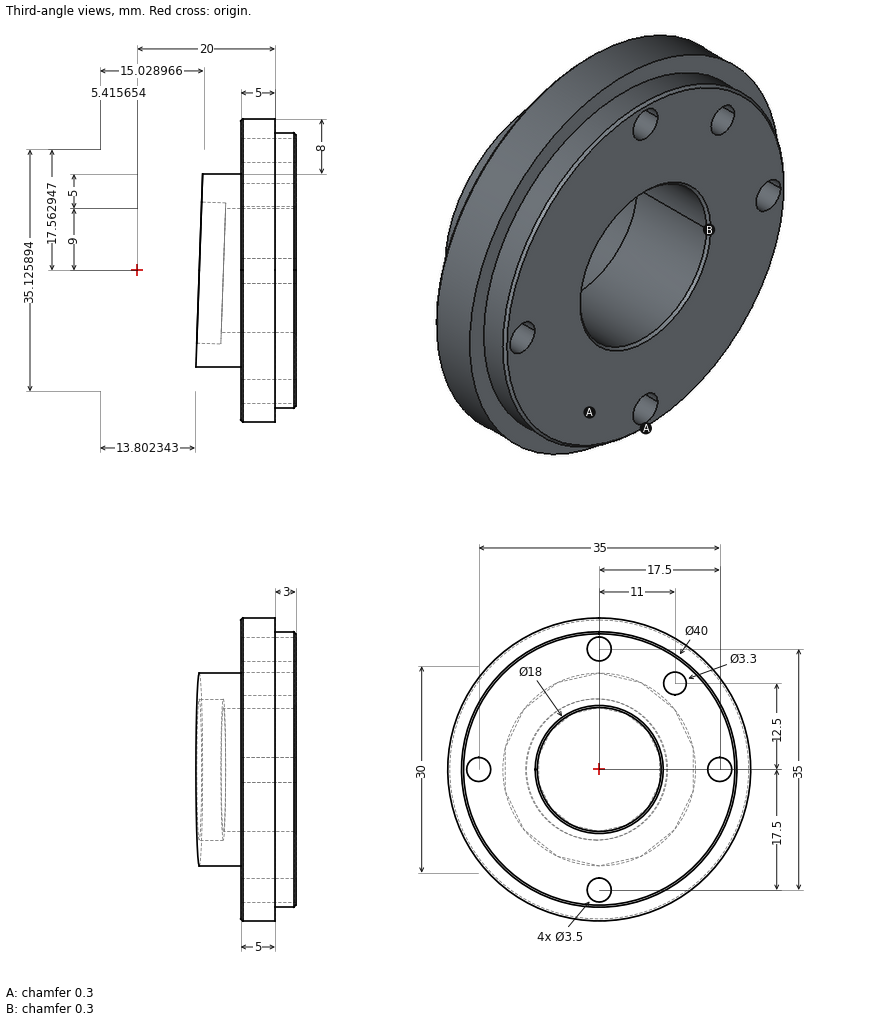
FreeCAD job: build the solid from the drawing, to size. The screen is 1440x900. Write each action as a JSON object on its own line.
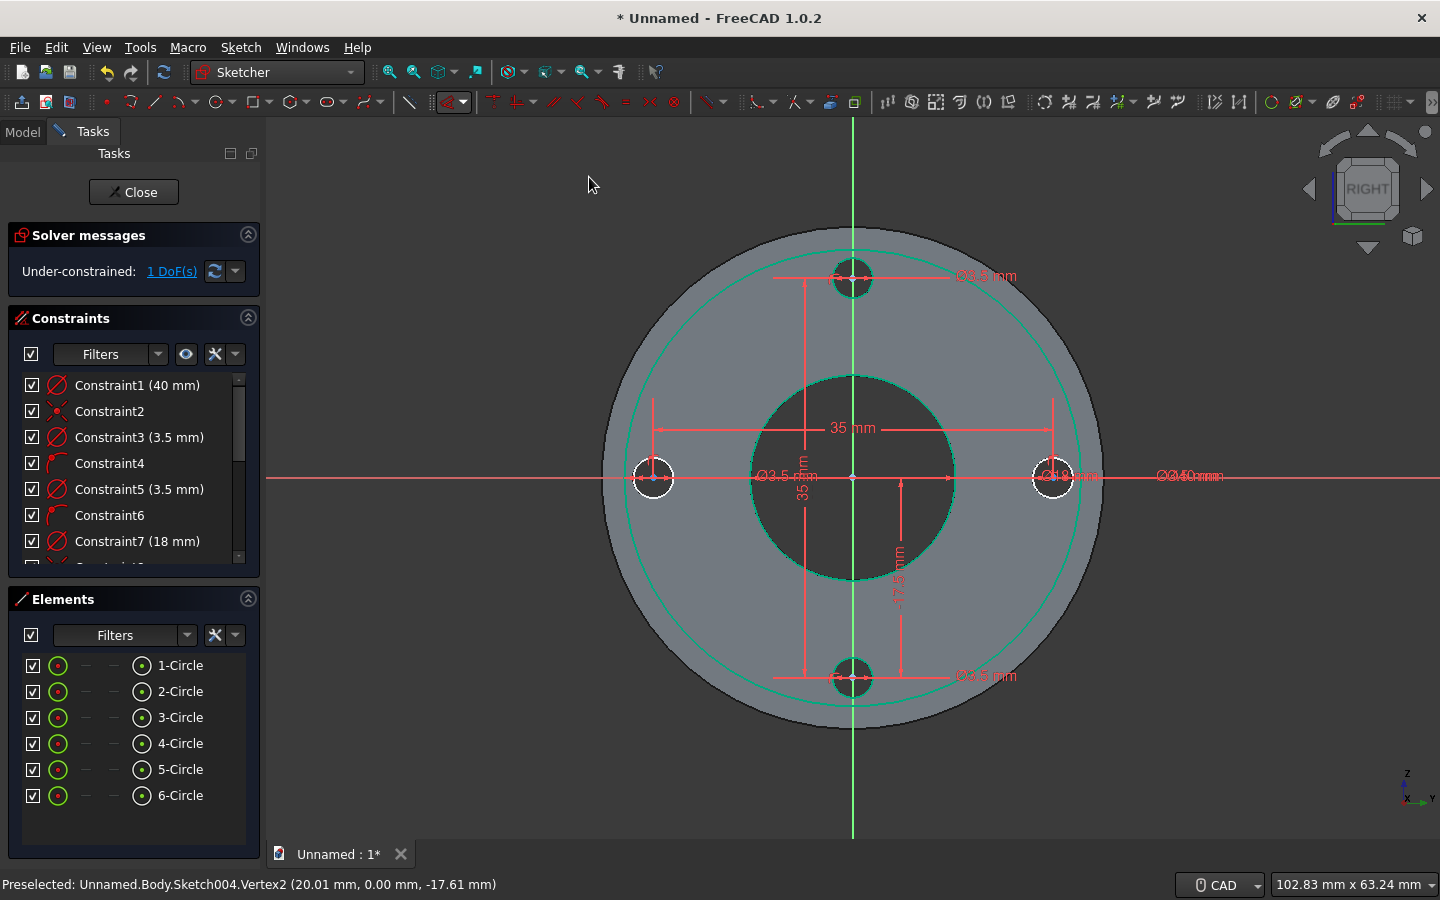
{"action": "left_click", "coordinate": [1053, 478]}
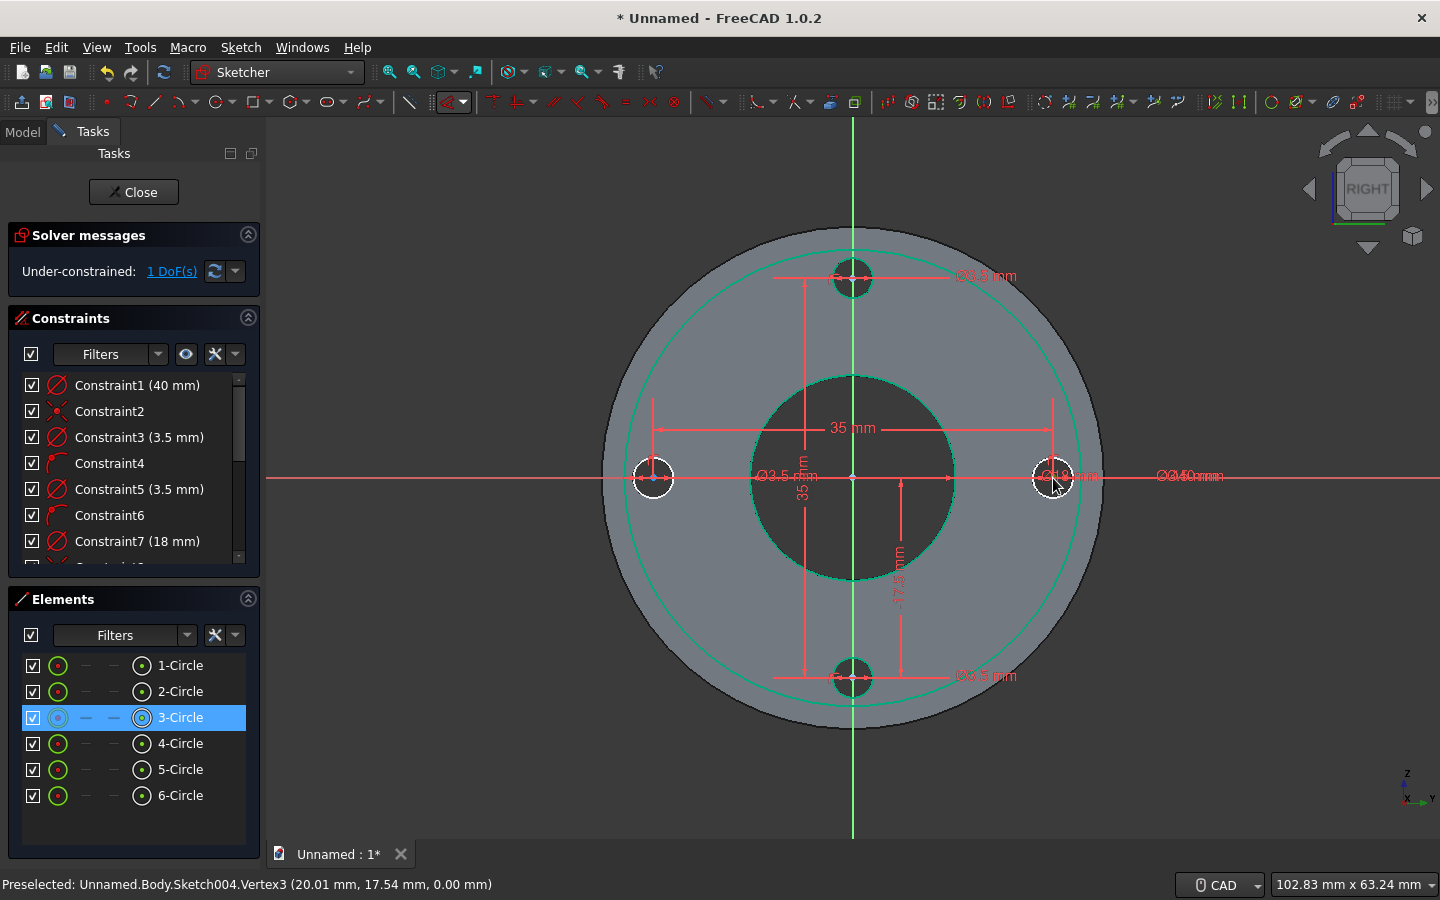
{"action": "key", "text": "l"}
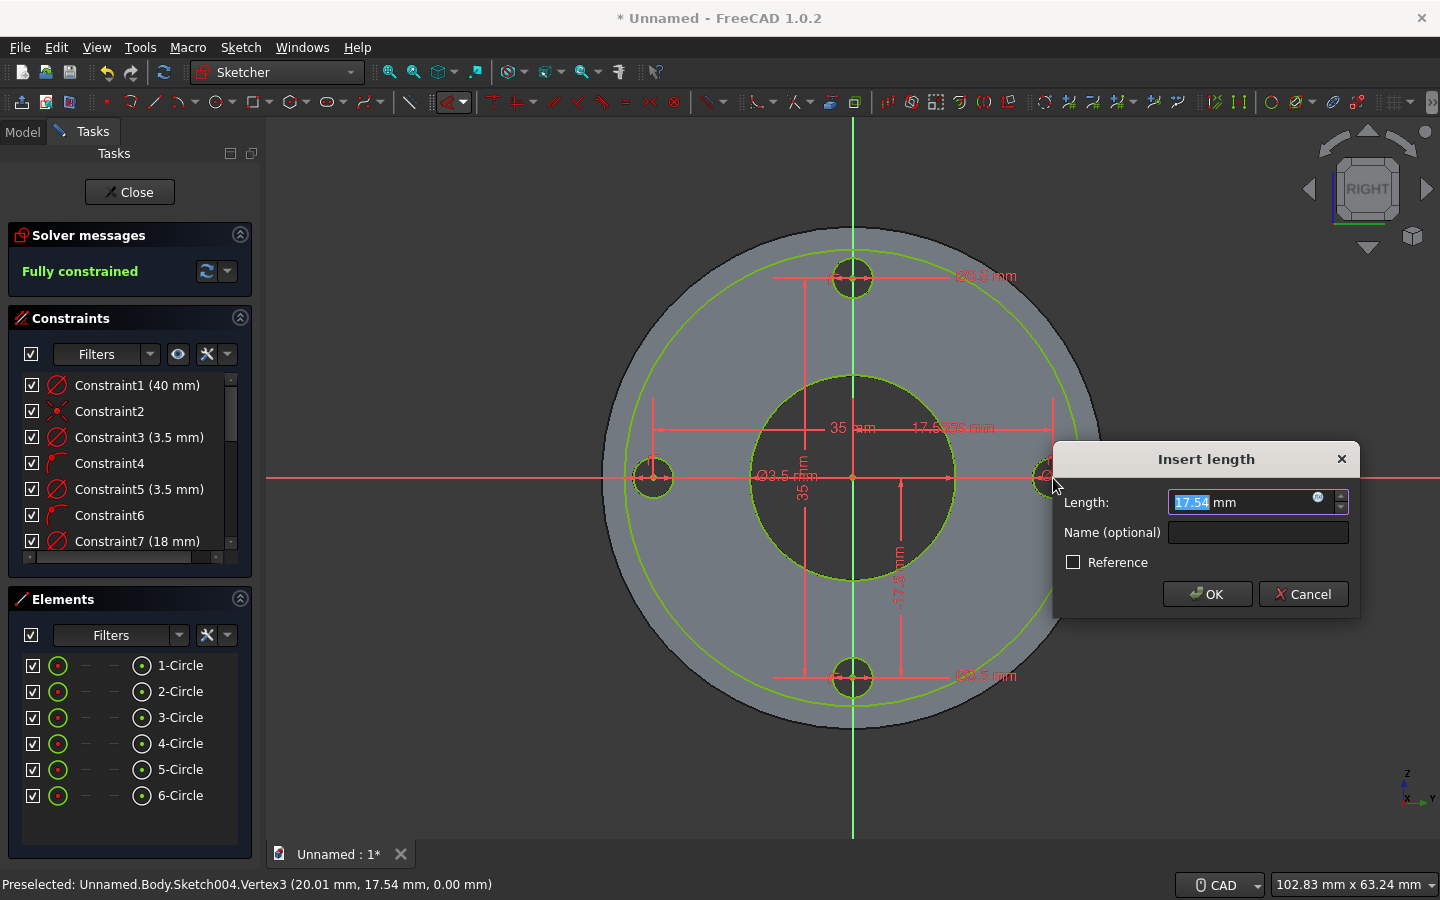
{"action": "type", "text": "17.5"}
{"action": "key", "text": "Return"}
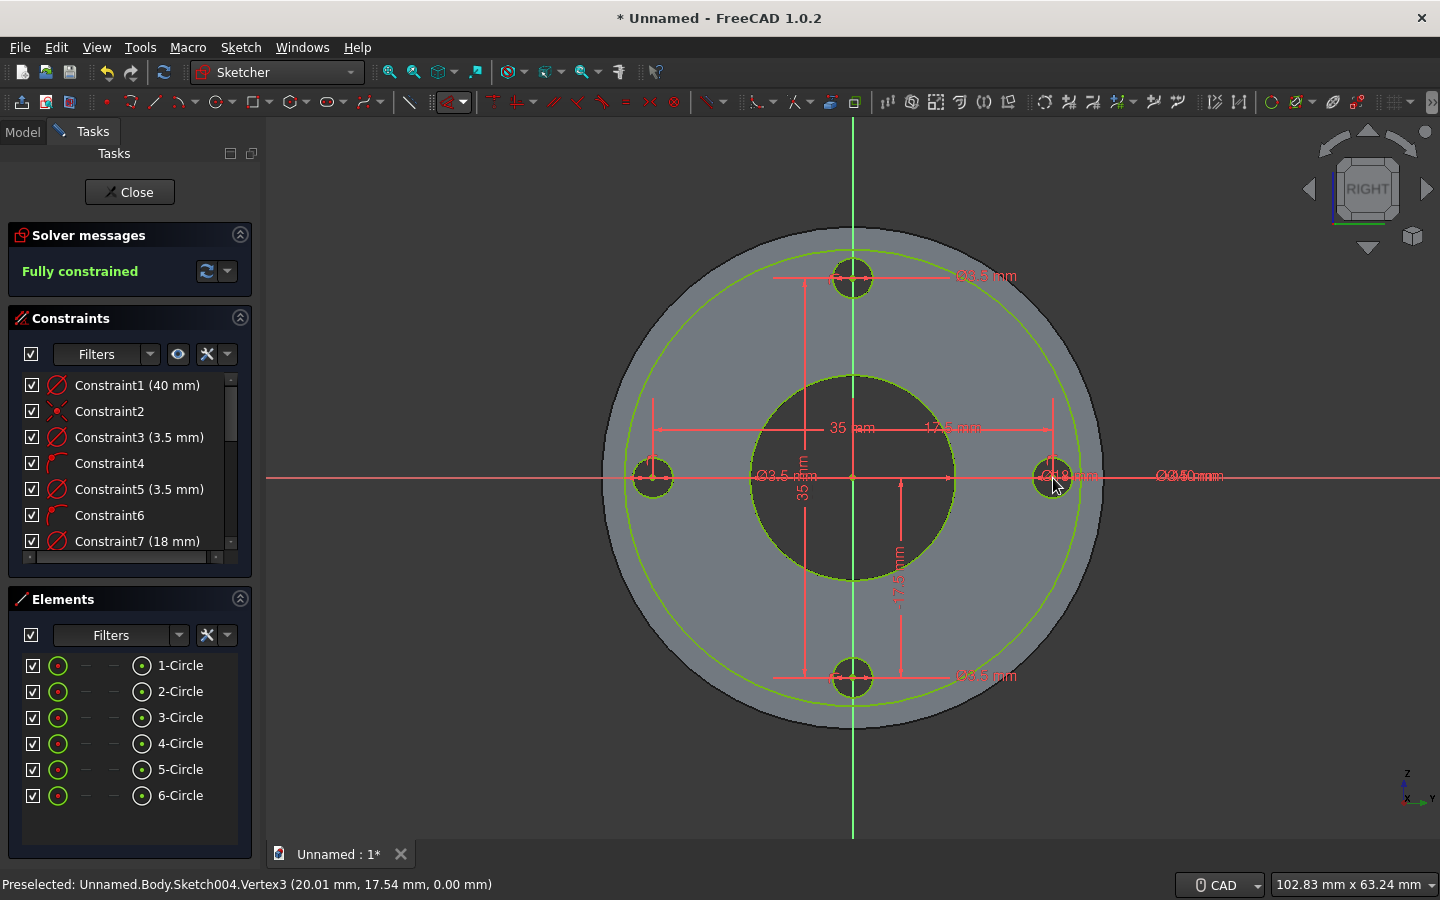
{"action": "left_click", "coordinate": [130, 192]}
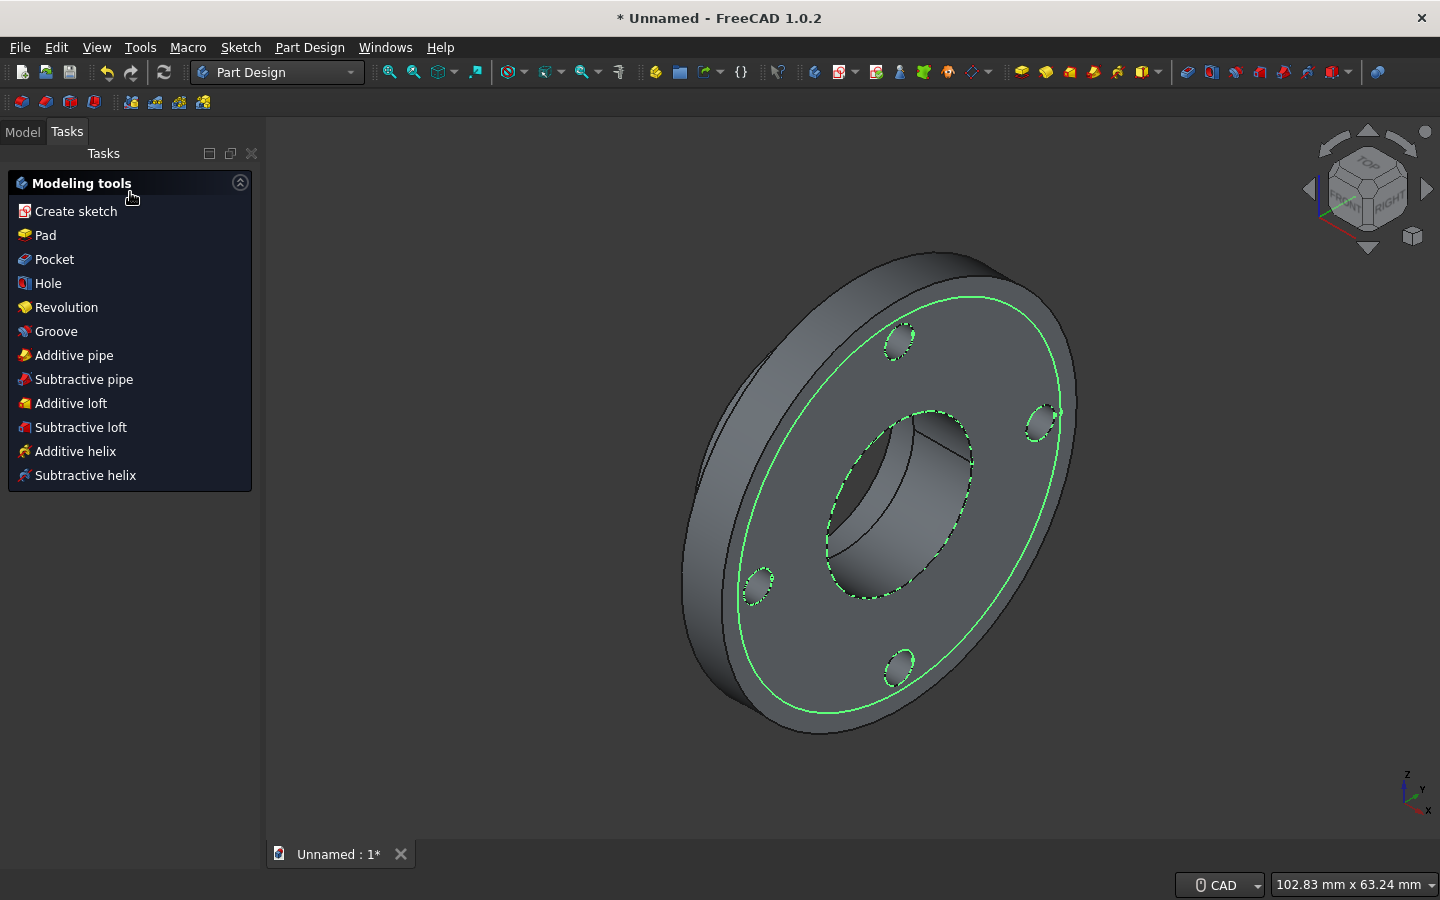
{"action": "left_click", "coordinate": [1022, 72]}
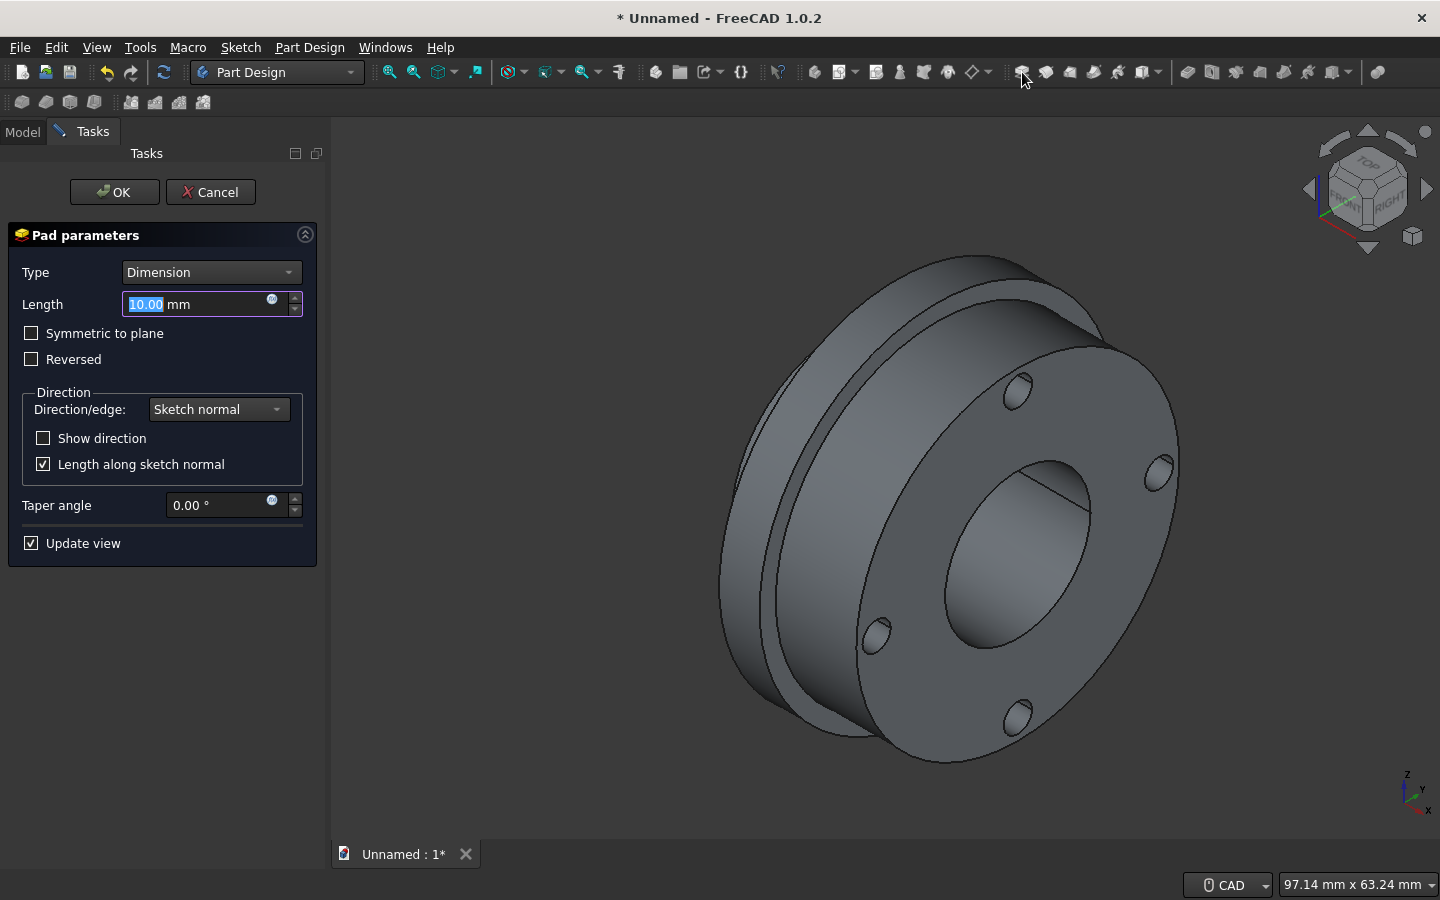
{"action": "type", "text": "3"}
{"action": "key", "text": "Tab"}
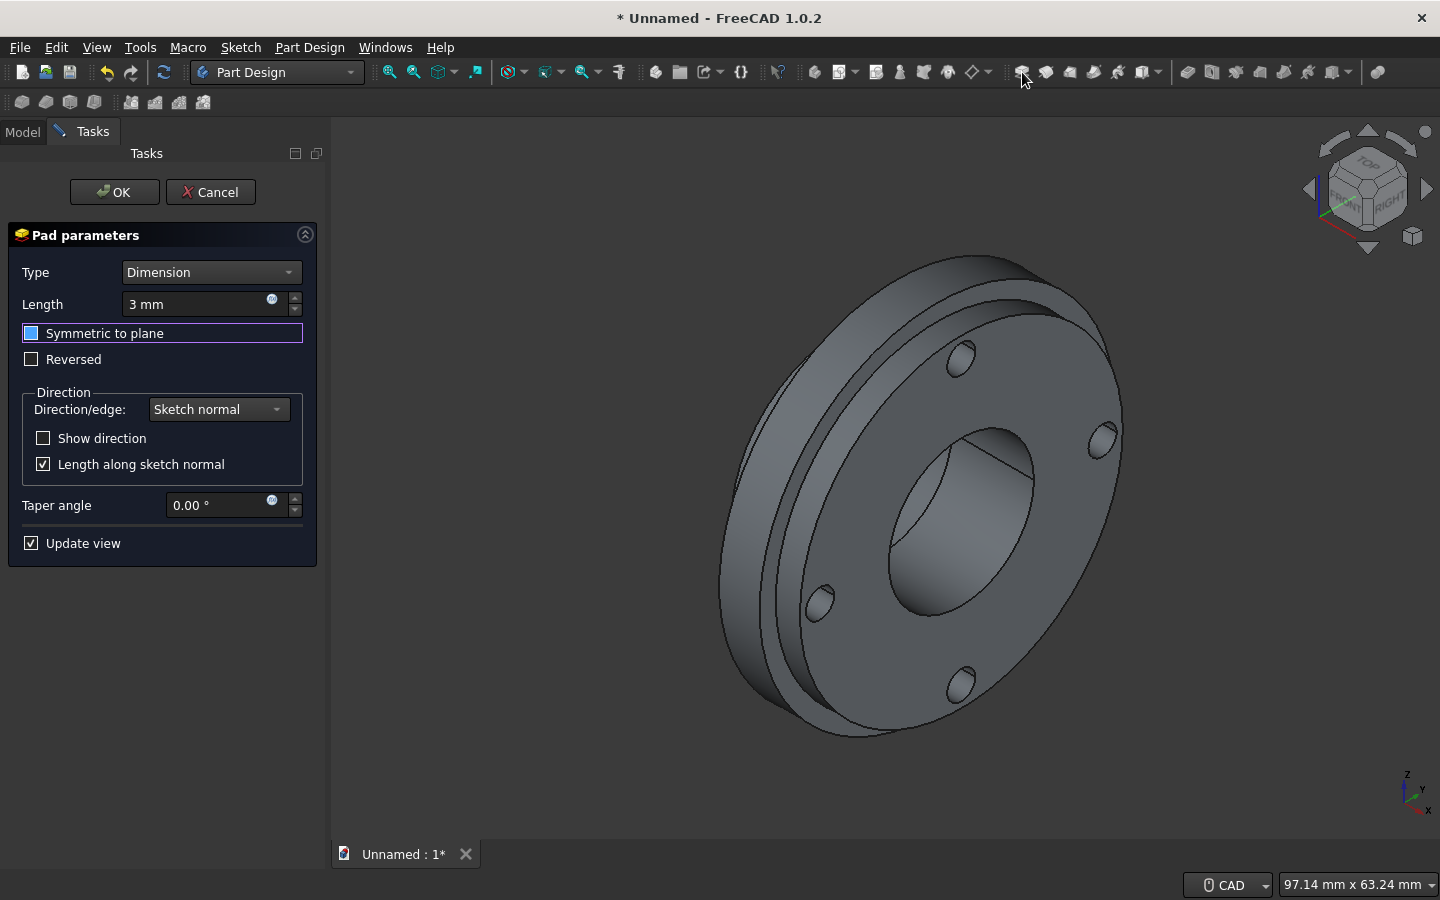
{"action": "left_click", "coordinate": [115, 192]}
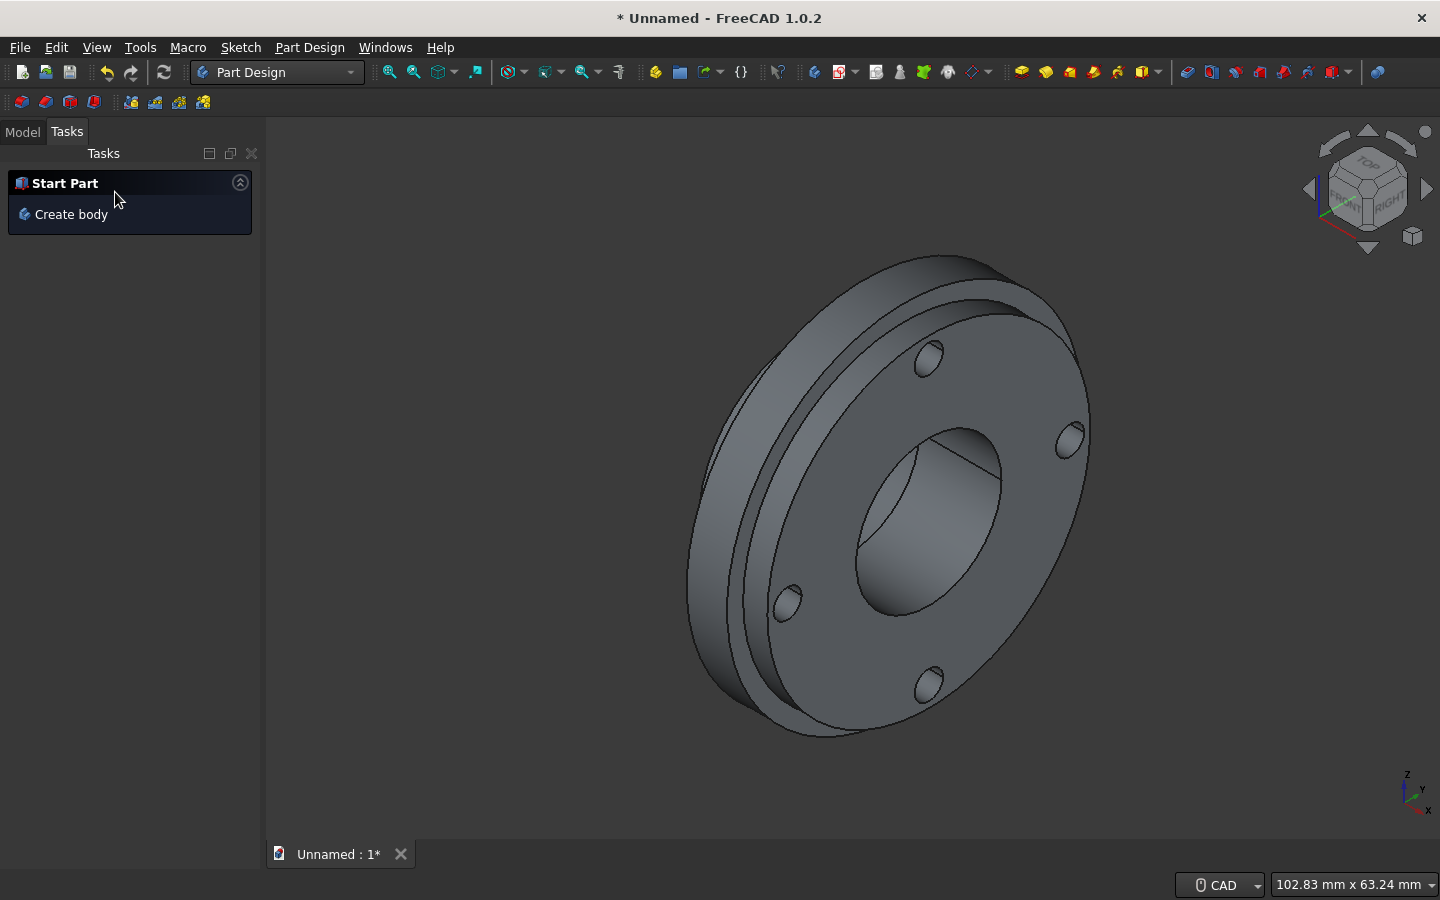
{"action": "left_click", "coordinate": [837, 681]}